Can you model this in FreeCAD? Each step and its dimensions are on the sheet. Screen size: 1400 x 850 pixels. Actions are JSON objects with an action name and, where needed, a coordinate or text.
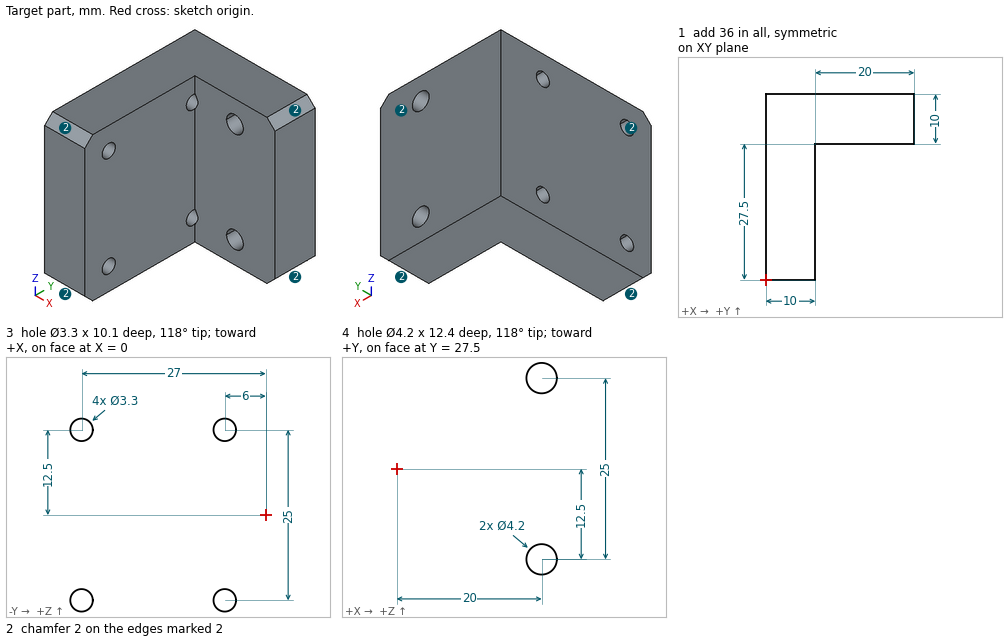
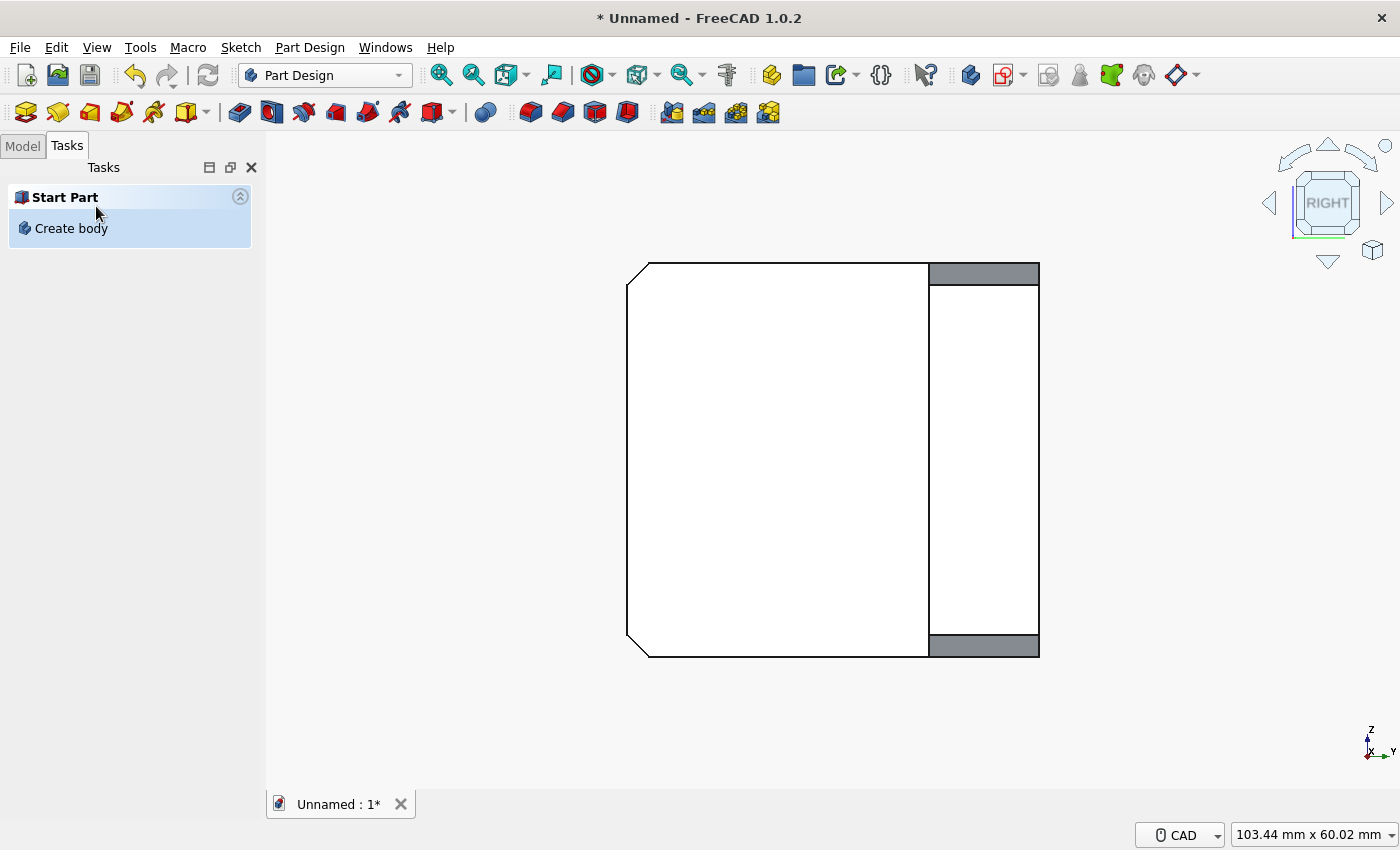
{"action": "key", "text": "6"}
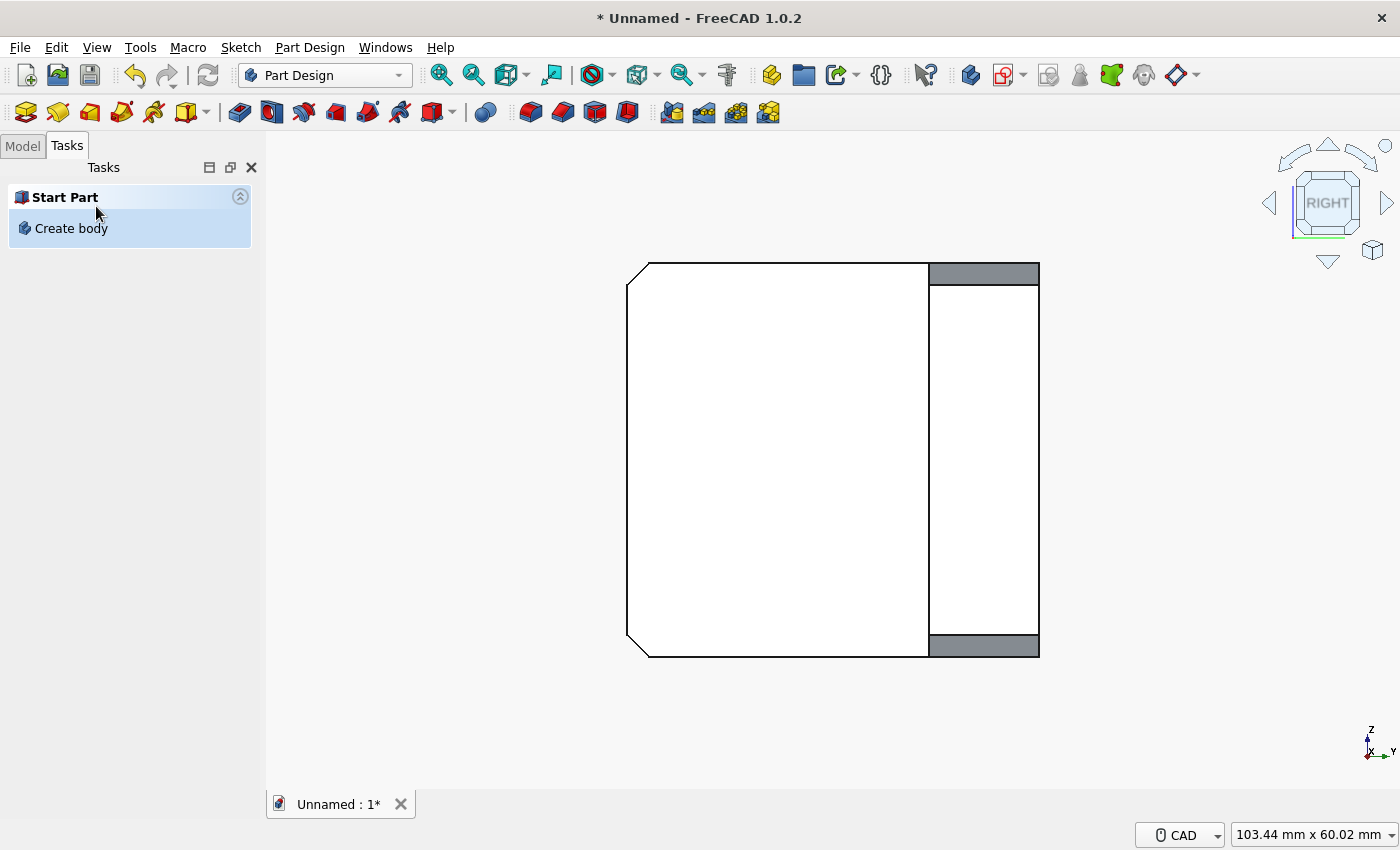
{"action": "left_click", "coordinate": [833, 459]}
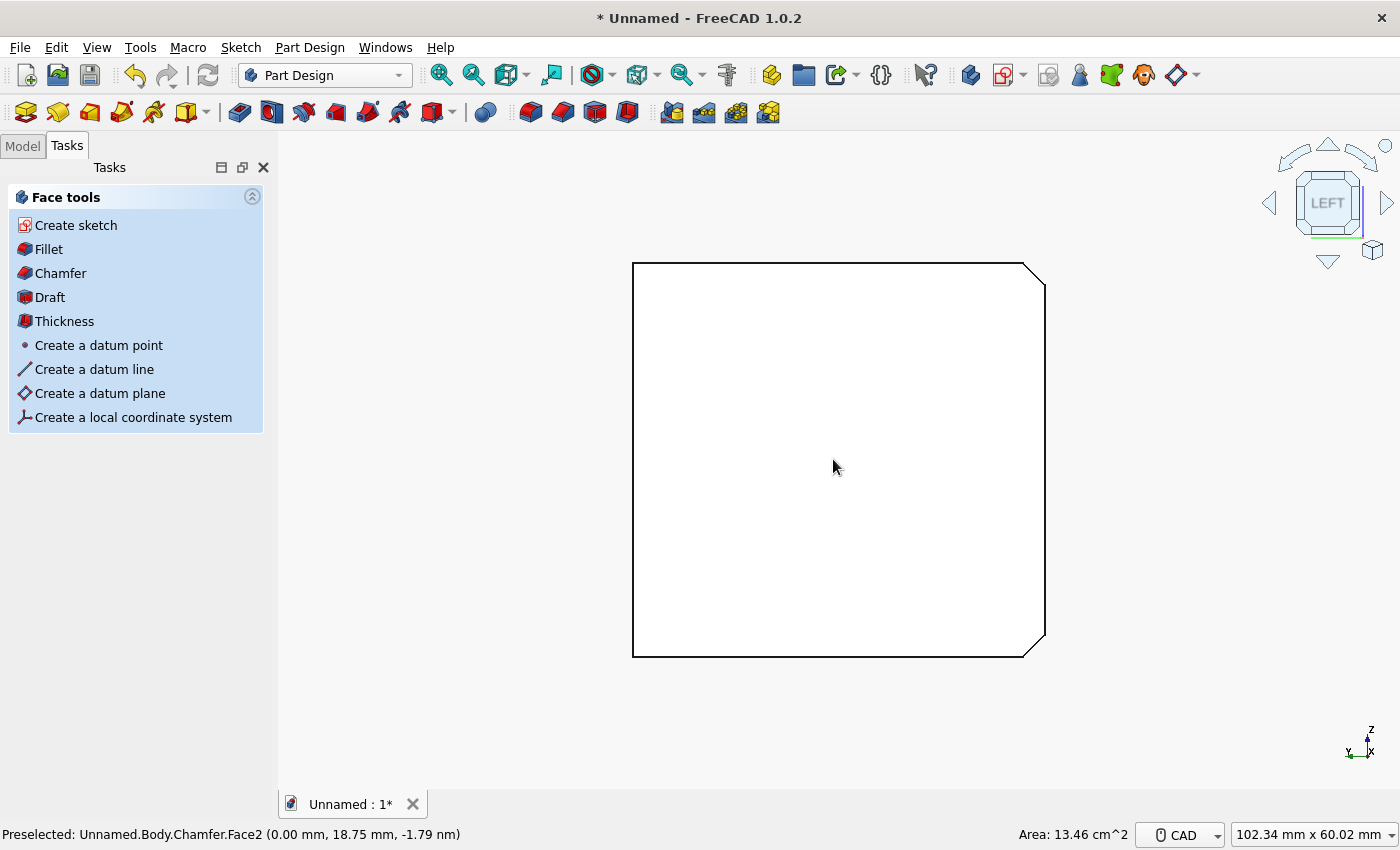
{"action": "left_click", "coordinate": [1004, 76]}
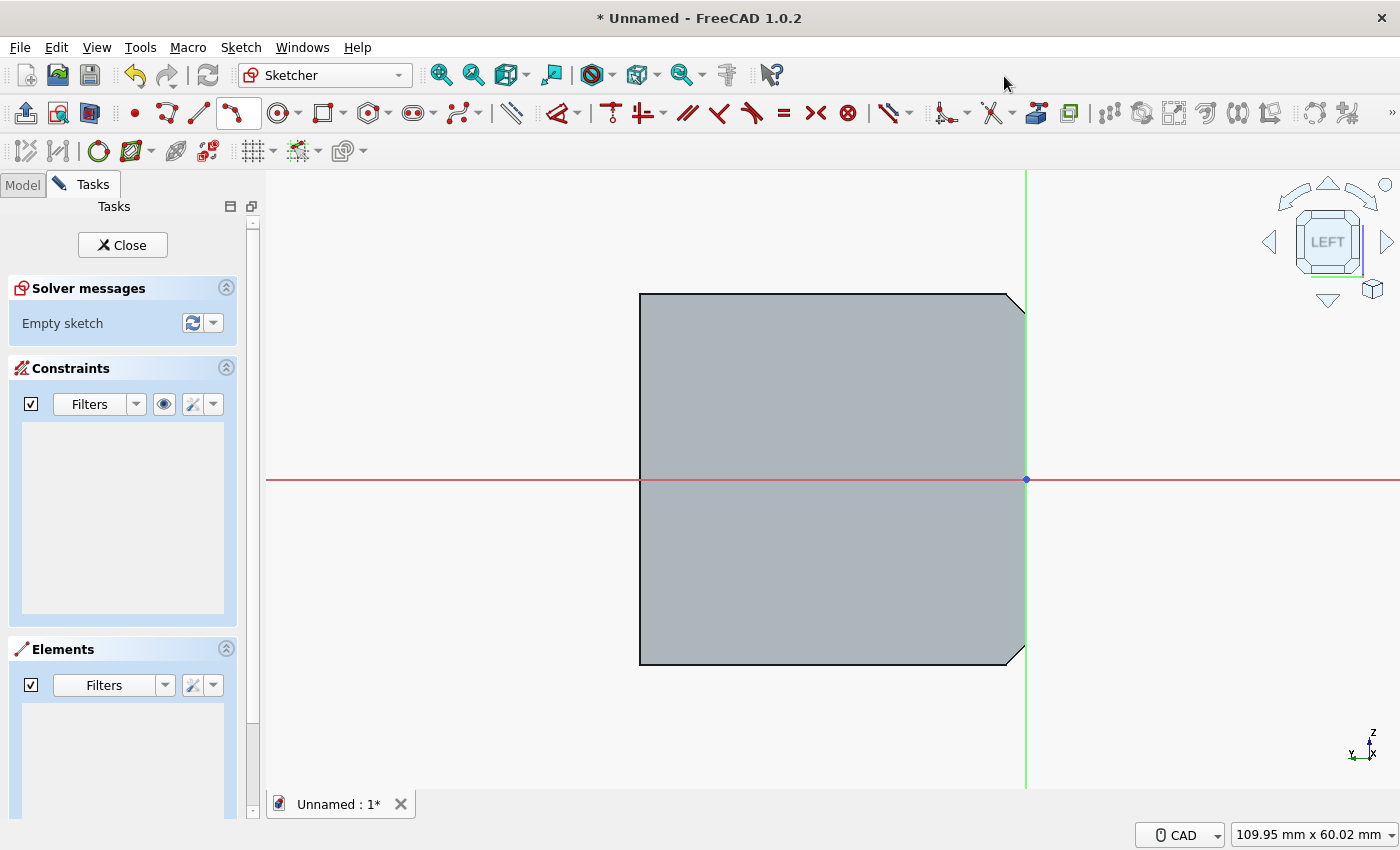
{"action": "scroll", "coordinate": [1111, 479], "scroll_direction": "up", "scroll_amount": 2}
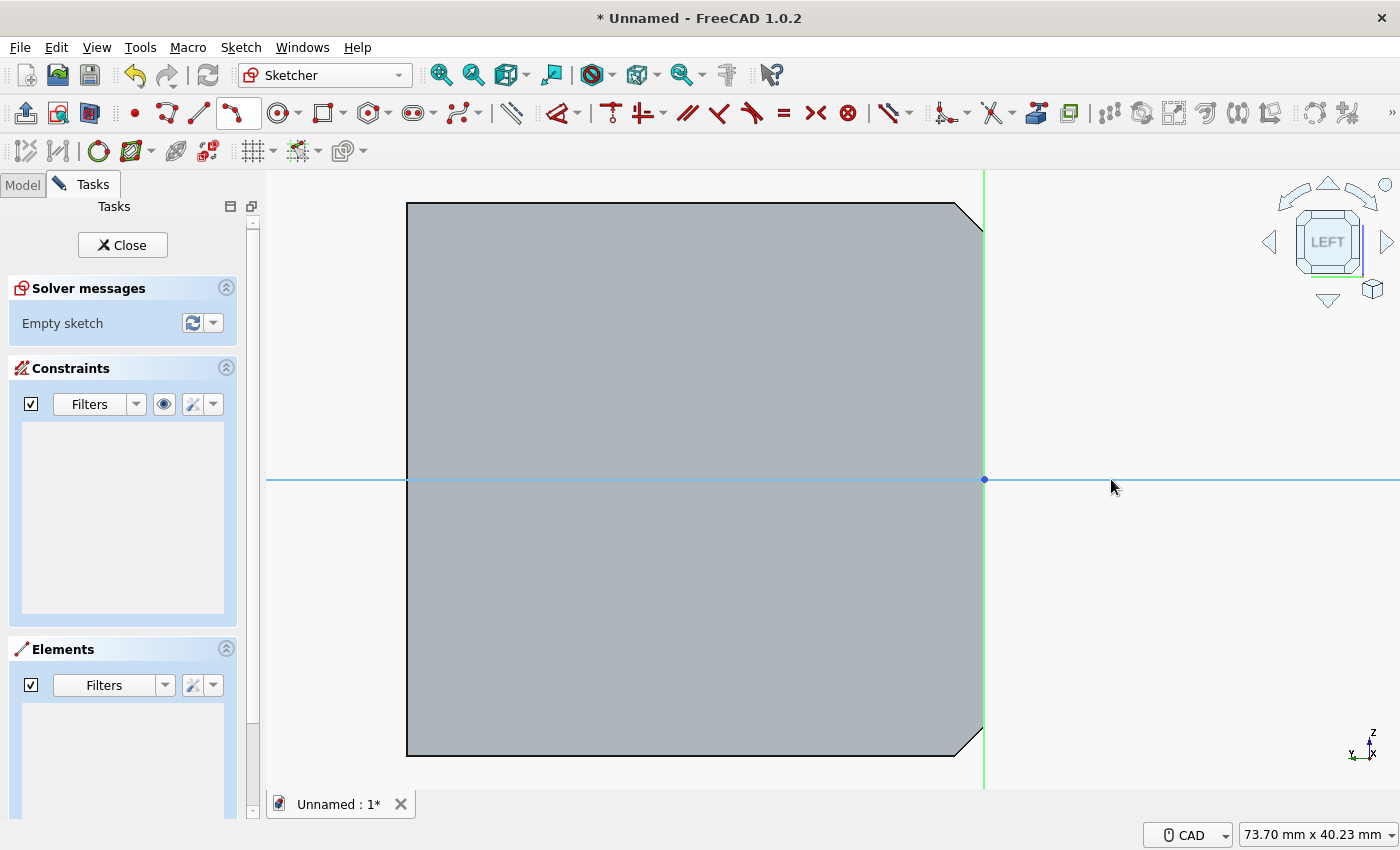
{"action": "key", "text": "g c"}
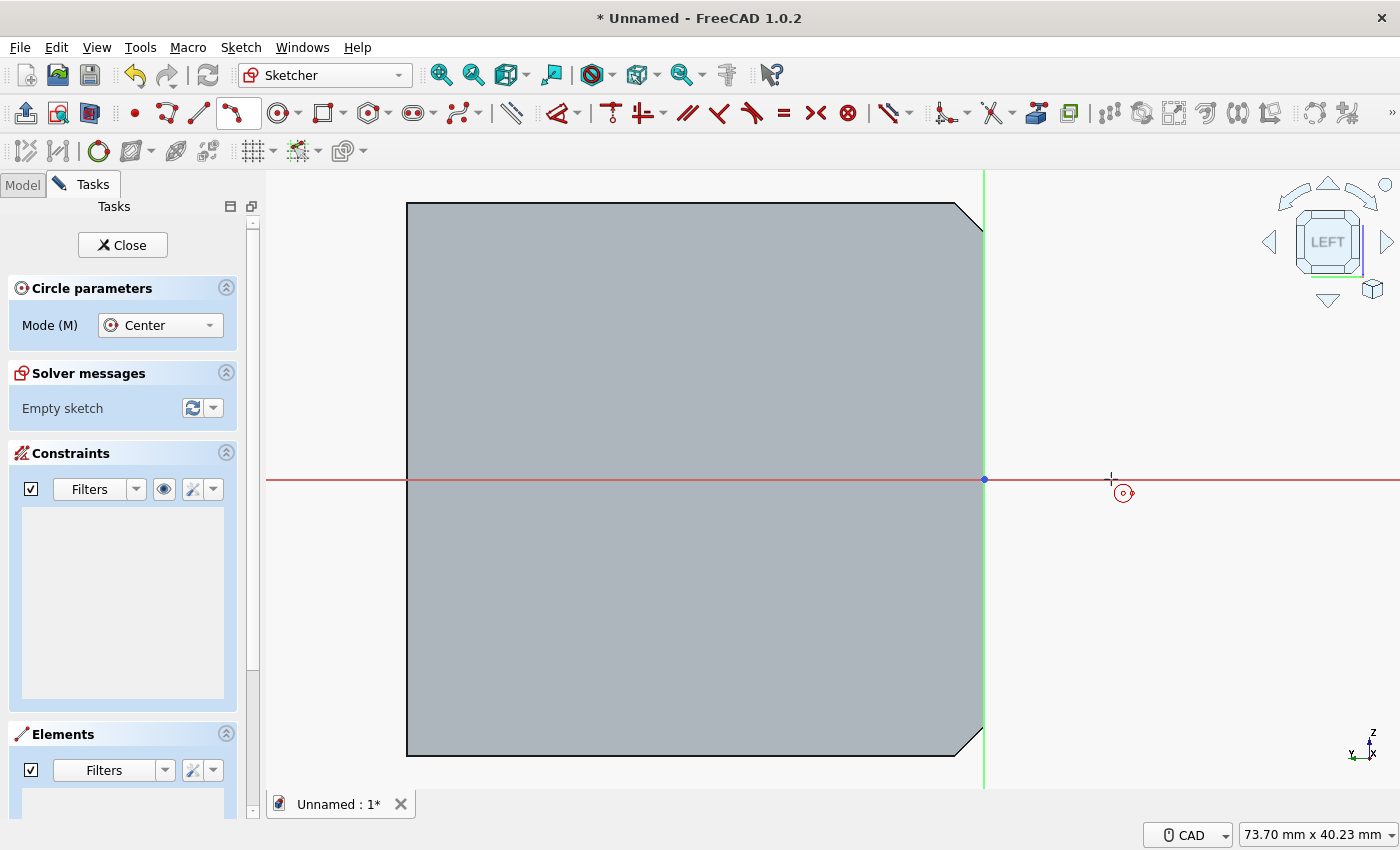
{"action": "left_click", "coordinate": [569, 287]}
{"action": "left_click", "coordinate": [587, 269]}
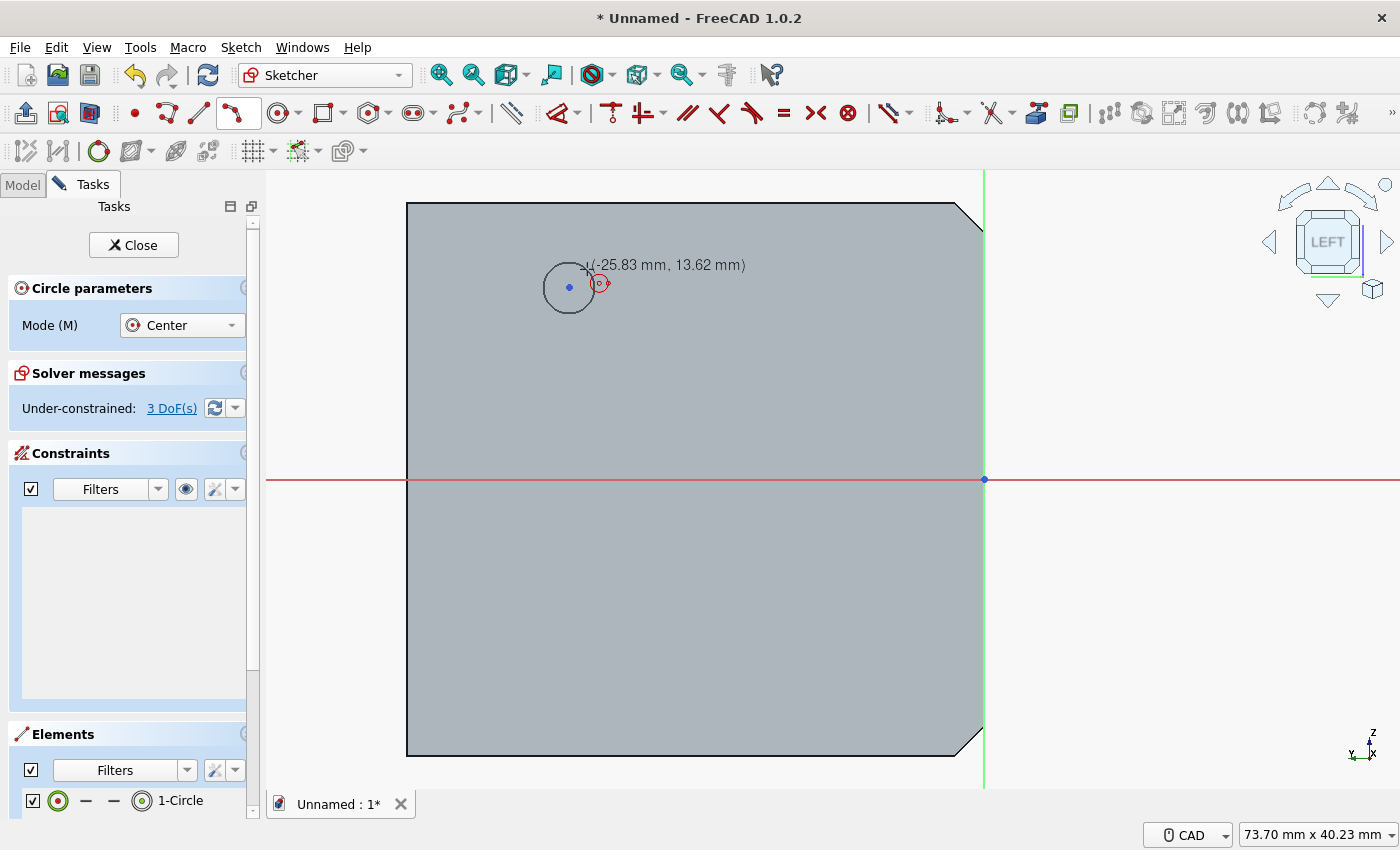
{"action": "left_click", "coordinate": [892, 287]}
{"action": "left_click", "coordinate": [910, 269]}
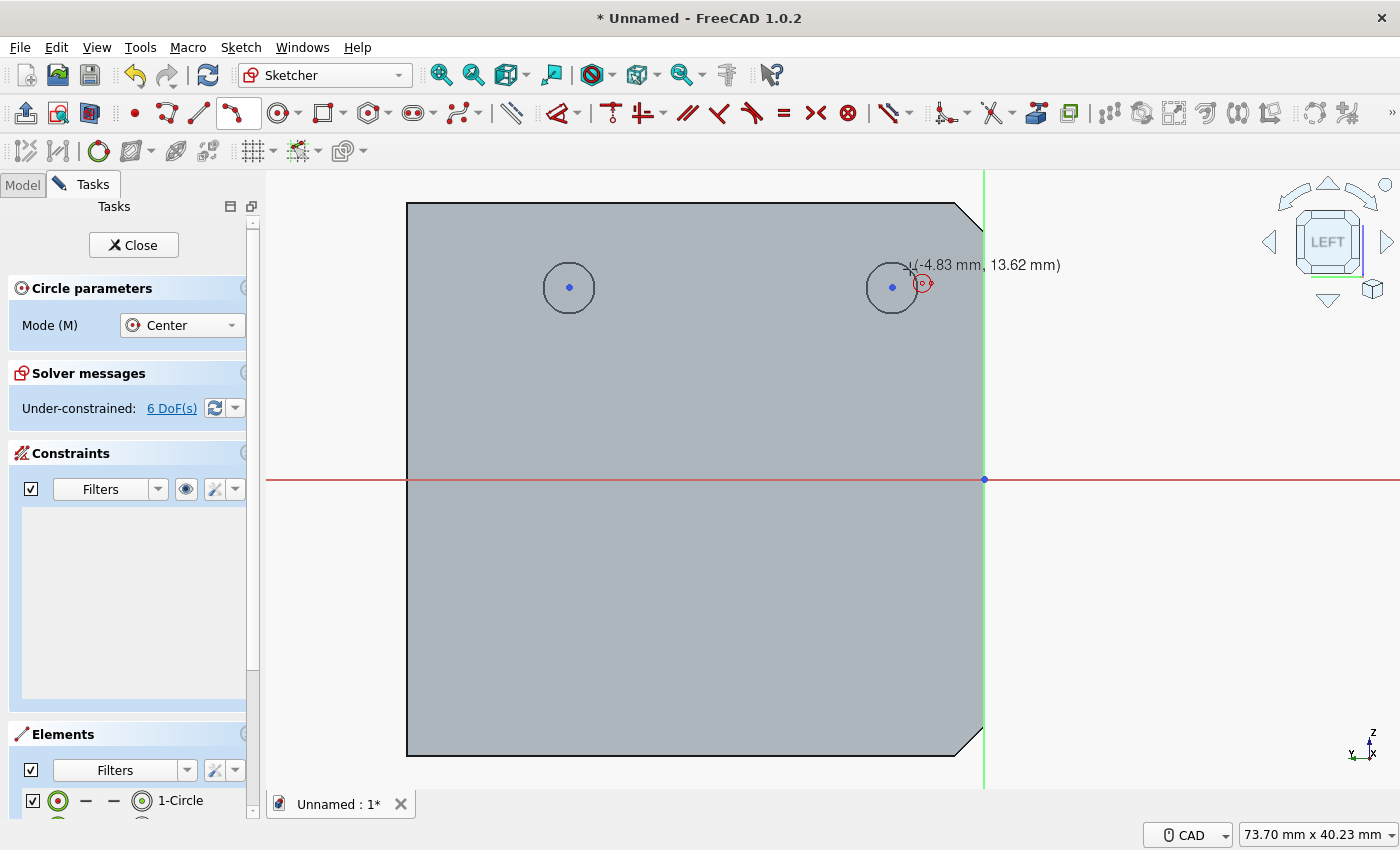
{"action": "left_click", "coordinate": [892, 672]}
{"action": "left_click", "coordinate": [910, 654]}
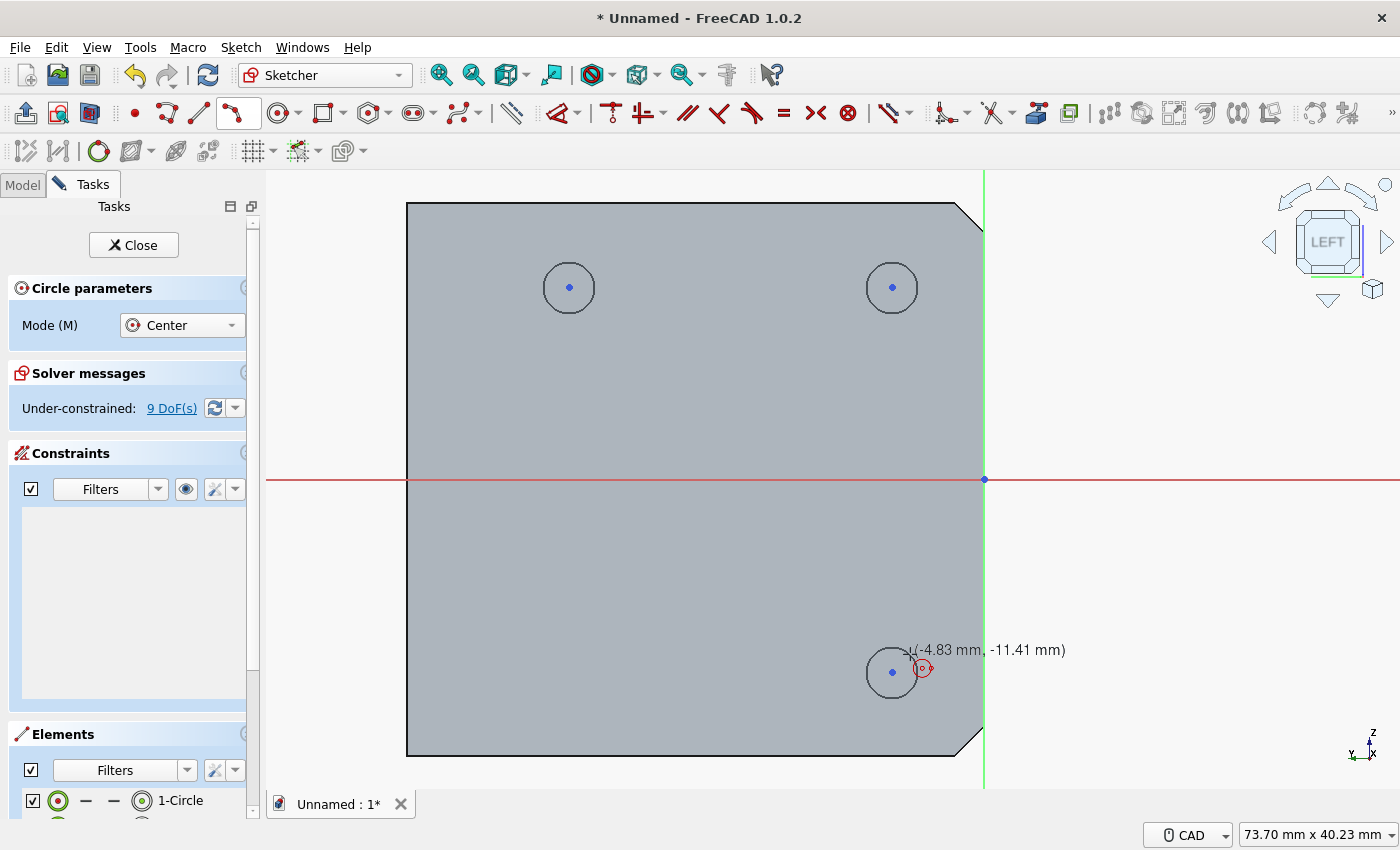
{"action": "left_click", "coordinate": [569, 672]}
{"action": "left_click", "coordinate": [587, 654]}
{"action": "key", "text": "Escape"}